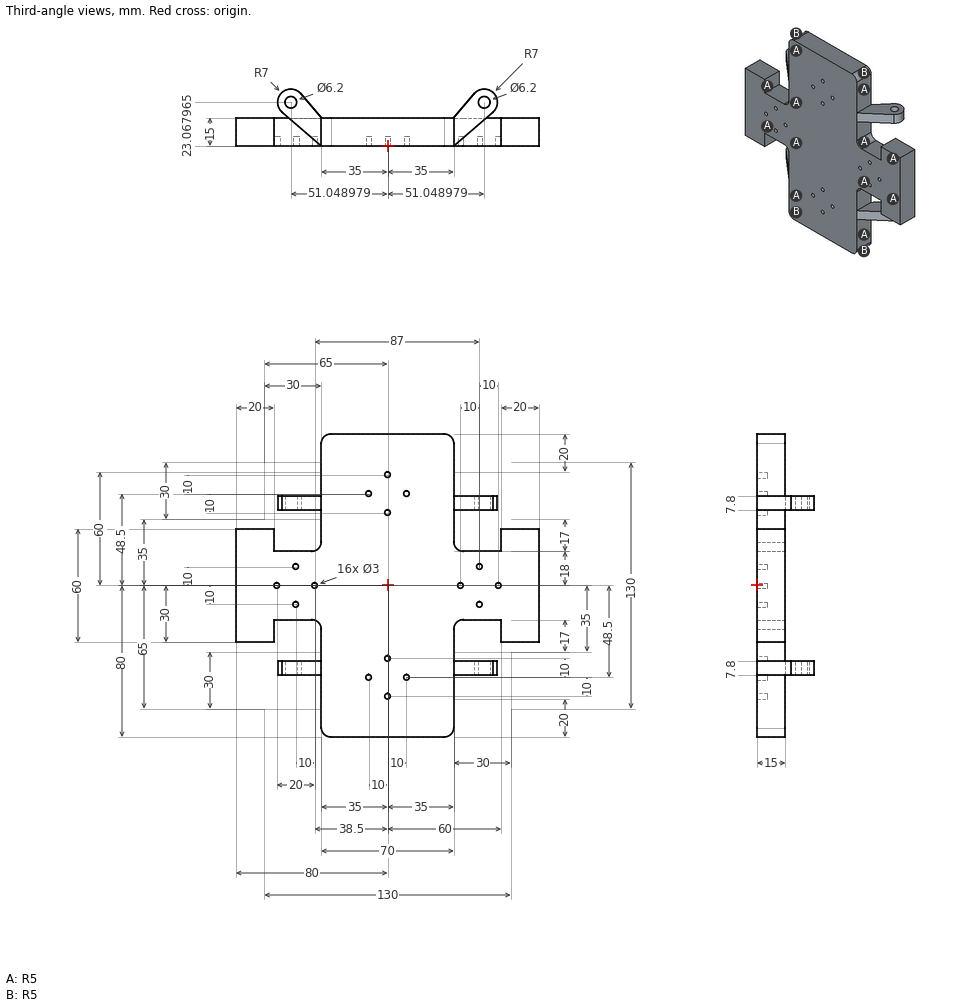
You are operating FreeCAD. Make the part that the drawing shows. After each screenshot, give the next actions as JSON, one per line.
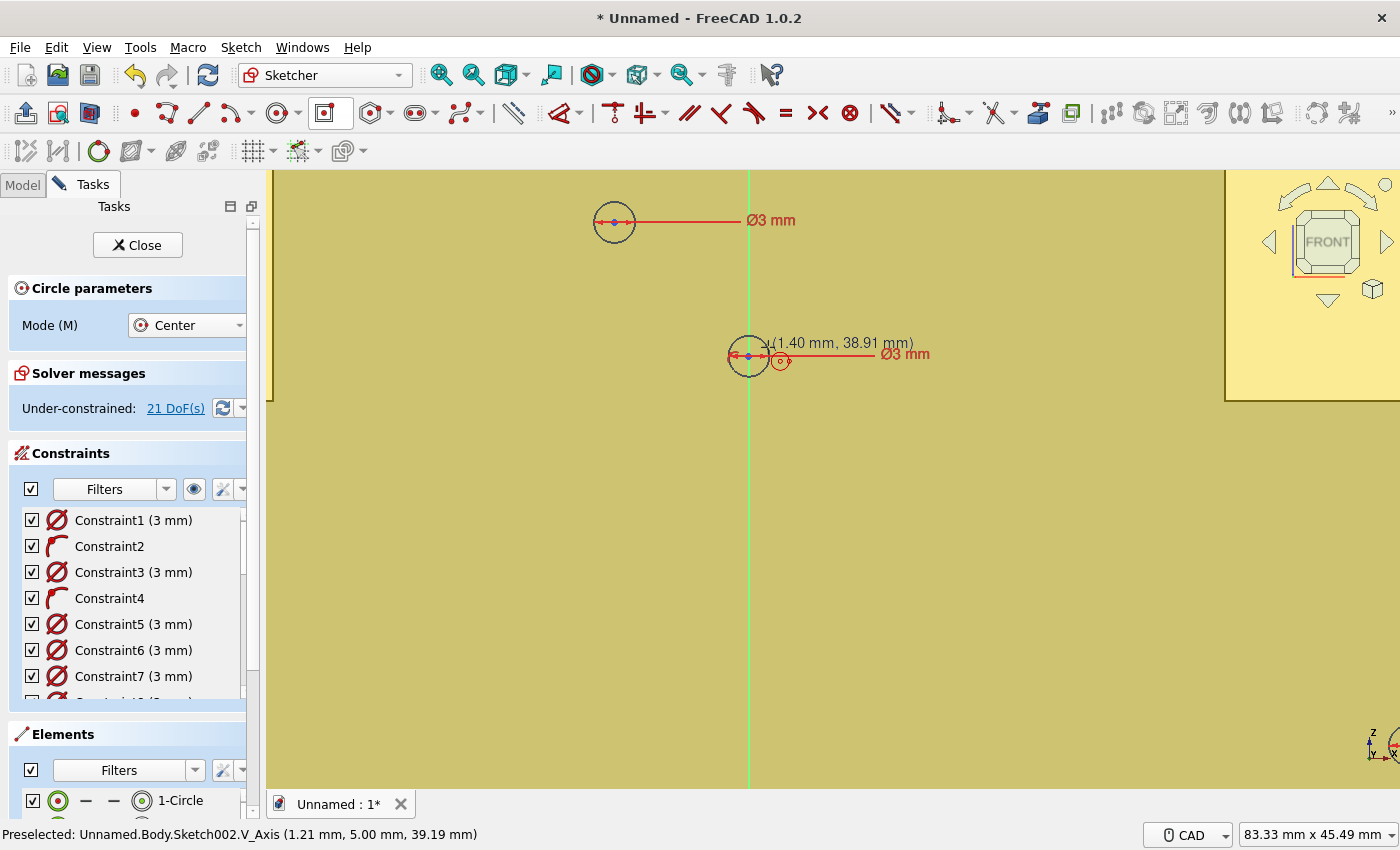
{"action": "scroll", "coordinate": [770, 349], "scroll_direction": "down", "scroll_amount": 7}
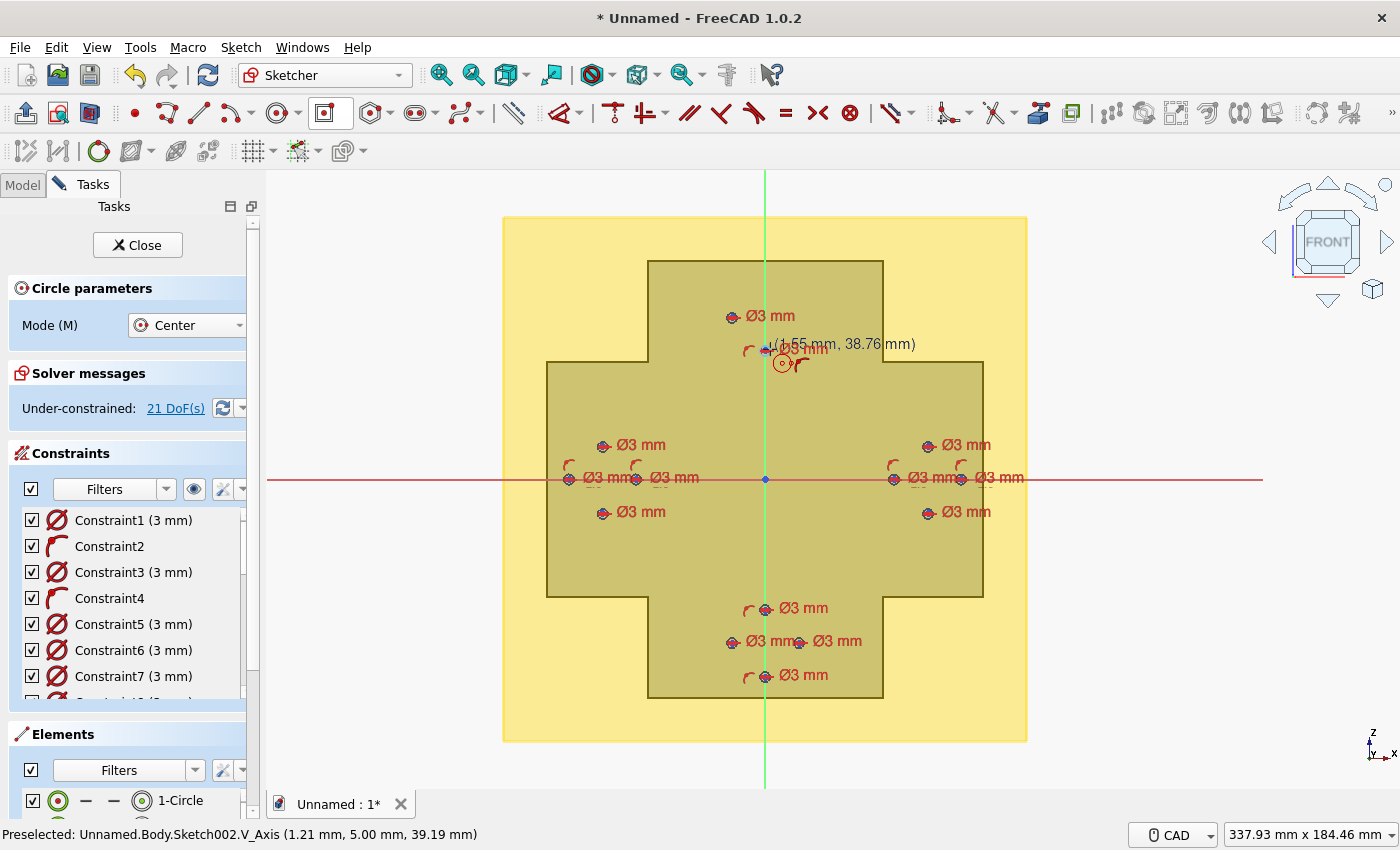
{"action": "left_click", "coordinate": [799, 317]}
{"action": "mouse_move", "coordinate": [802, 313]}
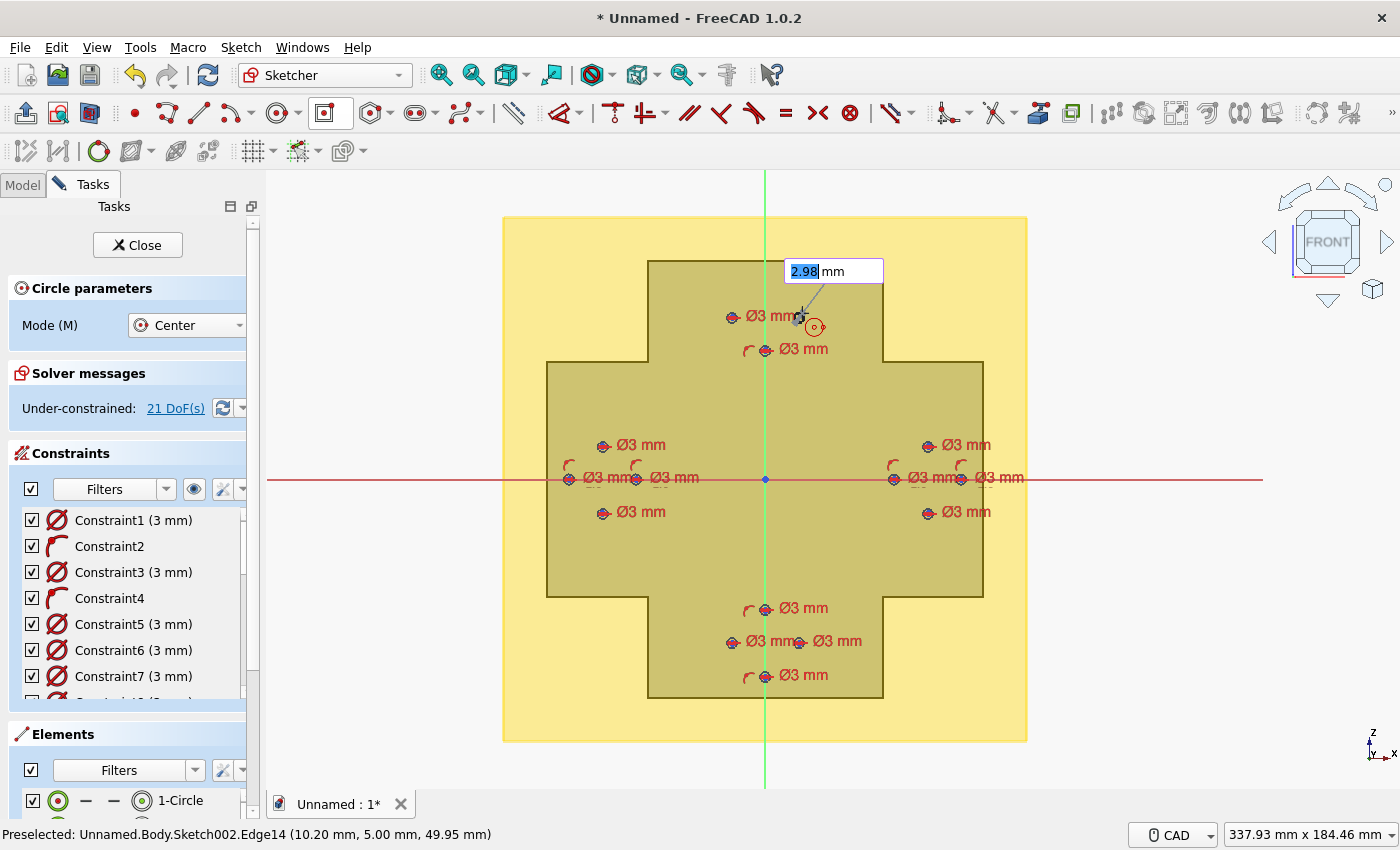
{"action": "type", "text": "3"}
{"action": "key", "text": "Return"}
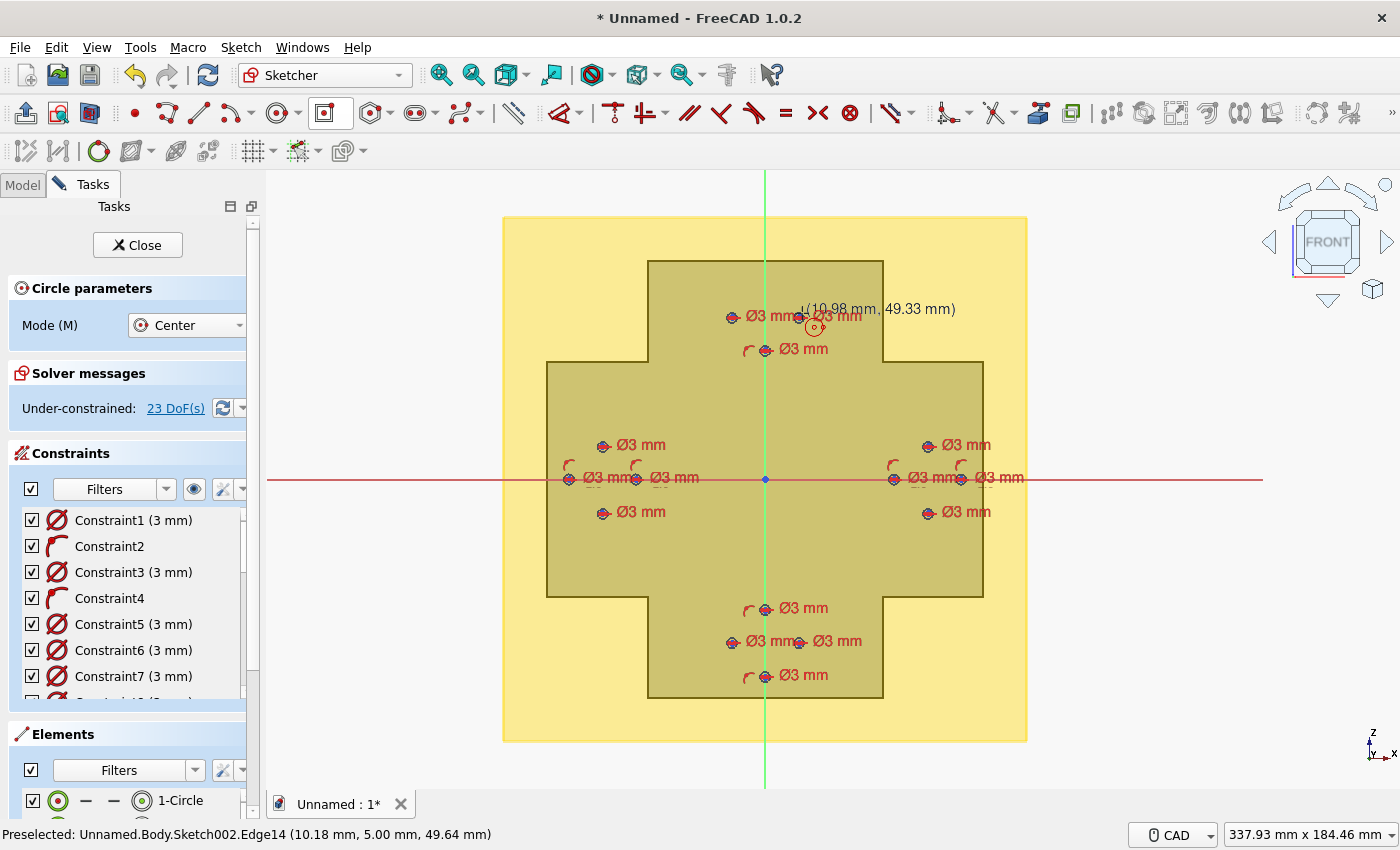
{"action": "scroll", "coordinate": [765, 283], "scroll_direction": "up", "scroll_amount": 8}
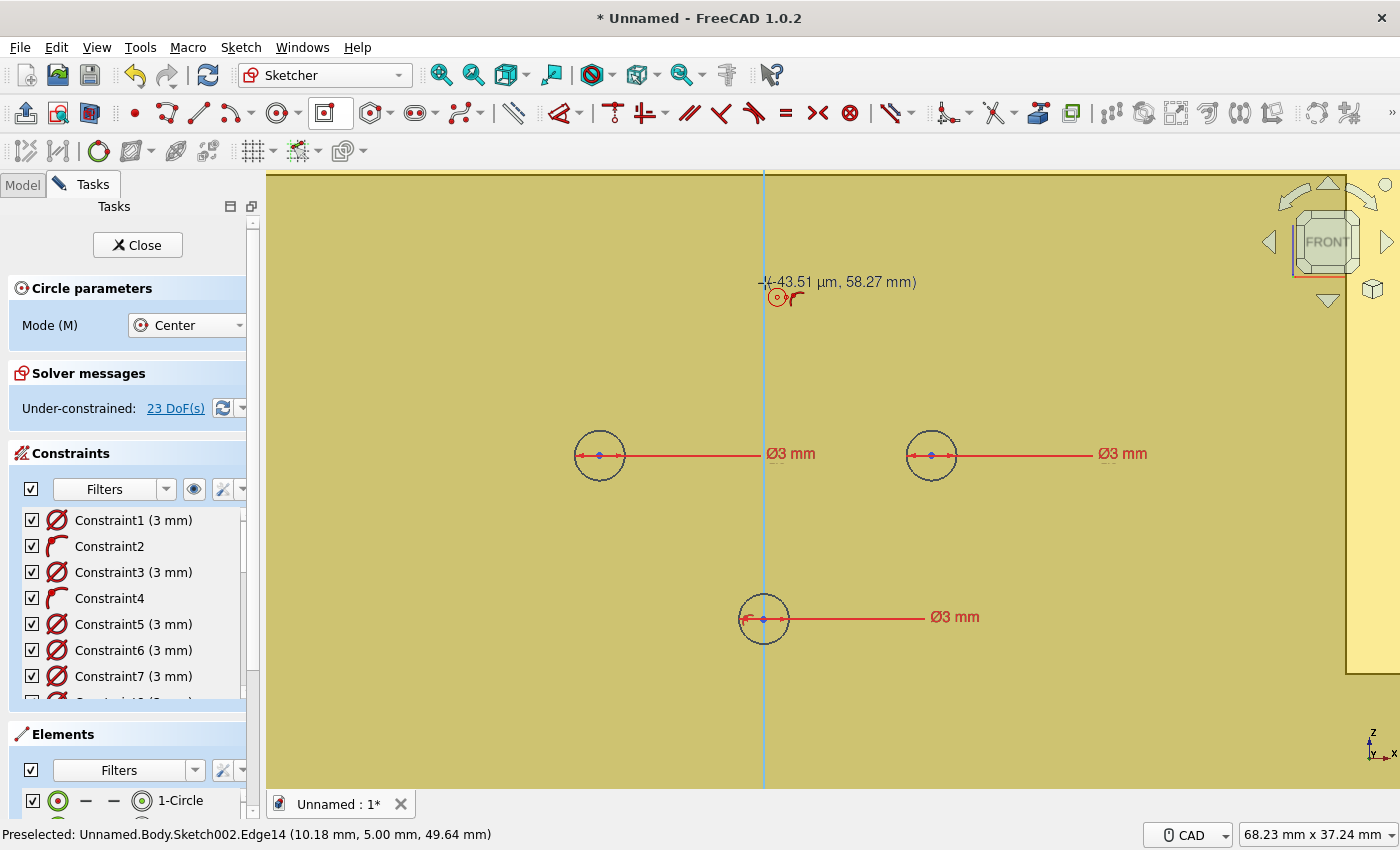
{"action": "scroll", "coordinate": [765, 283], "scroll_direction": "down", "scroll_amount": 8}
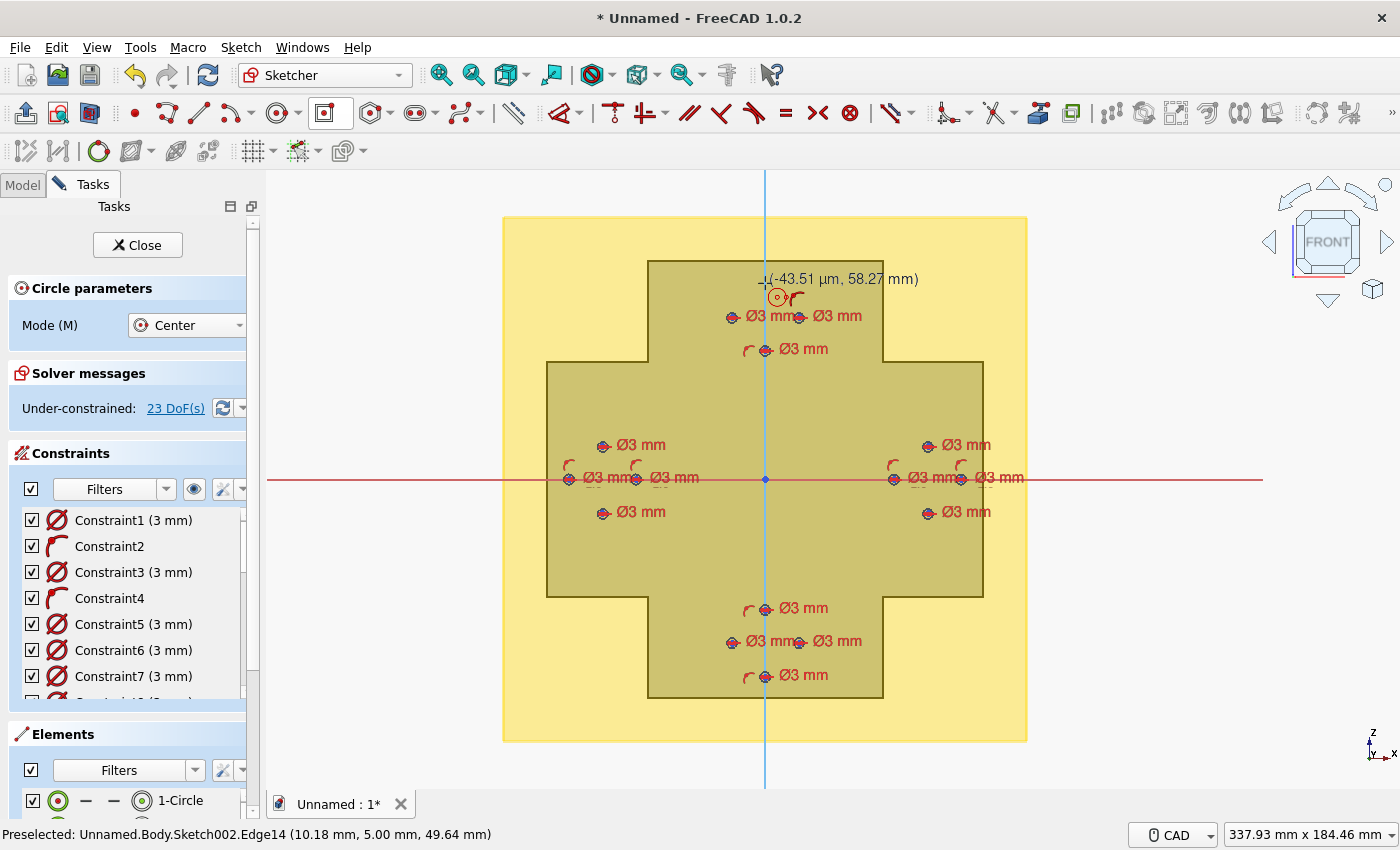
{"action": "left_click", "coordinate": [765, 283]}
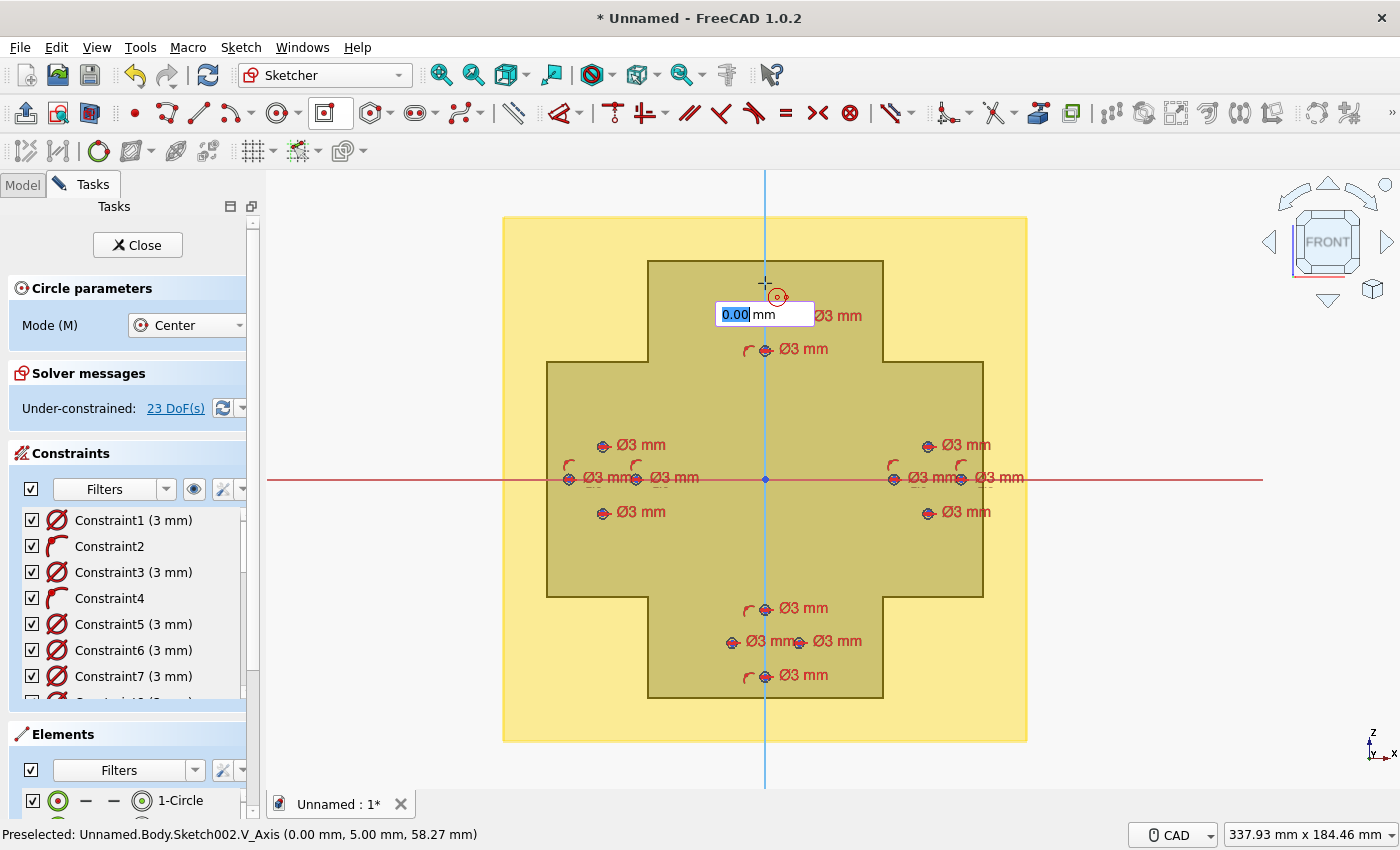
{"action": "scroll", "coordinate": [770, 282], "scroll_direction": "up", "scroll_amount": 7}
{"action": "mouse_move", "coordinate": [768, 279]}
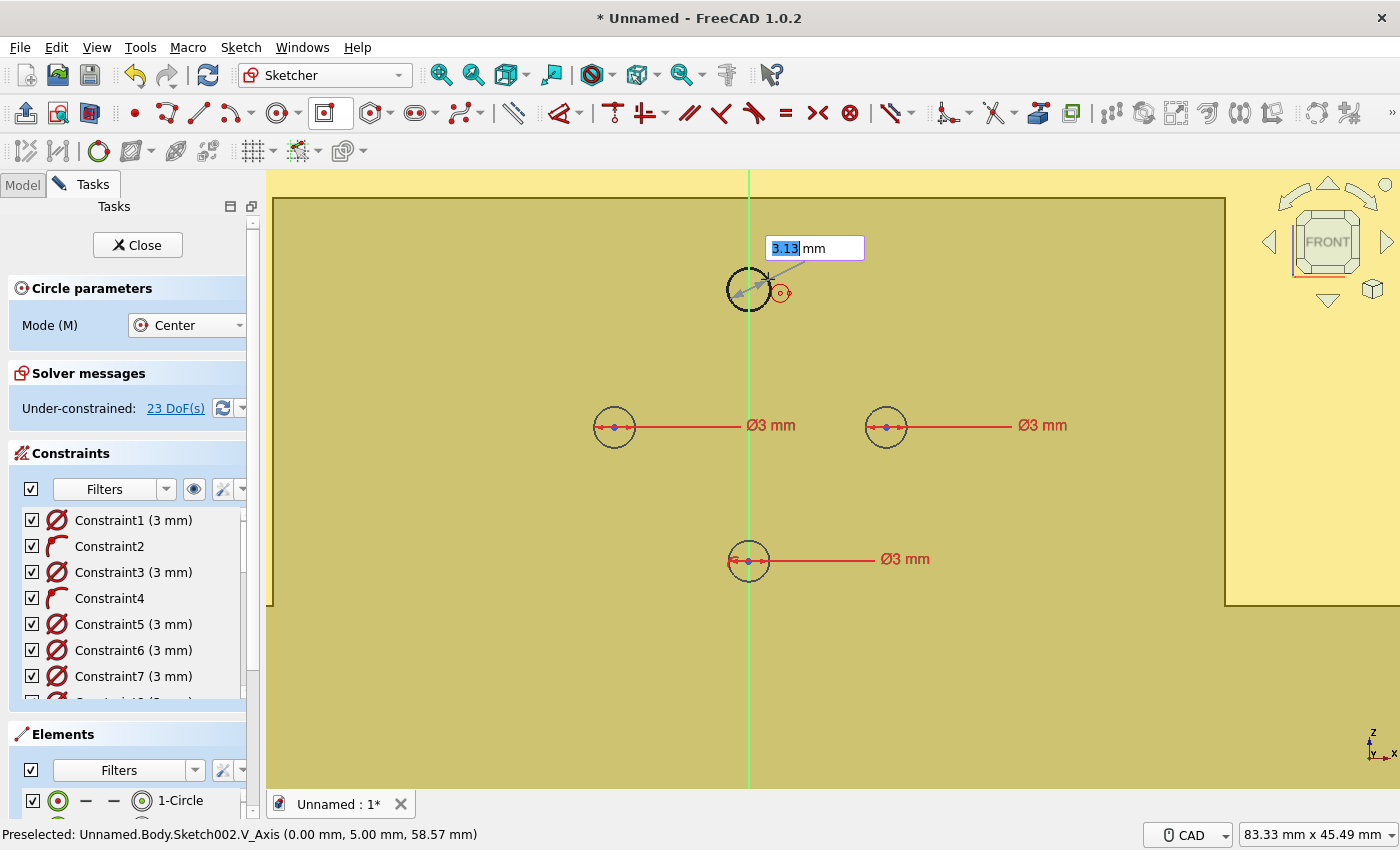
{"action": "type", "text": "3"}
{"action": "key", "text": "Return"}
{"action": "key", "text": "Escape"}